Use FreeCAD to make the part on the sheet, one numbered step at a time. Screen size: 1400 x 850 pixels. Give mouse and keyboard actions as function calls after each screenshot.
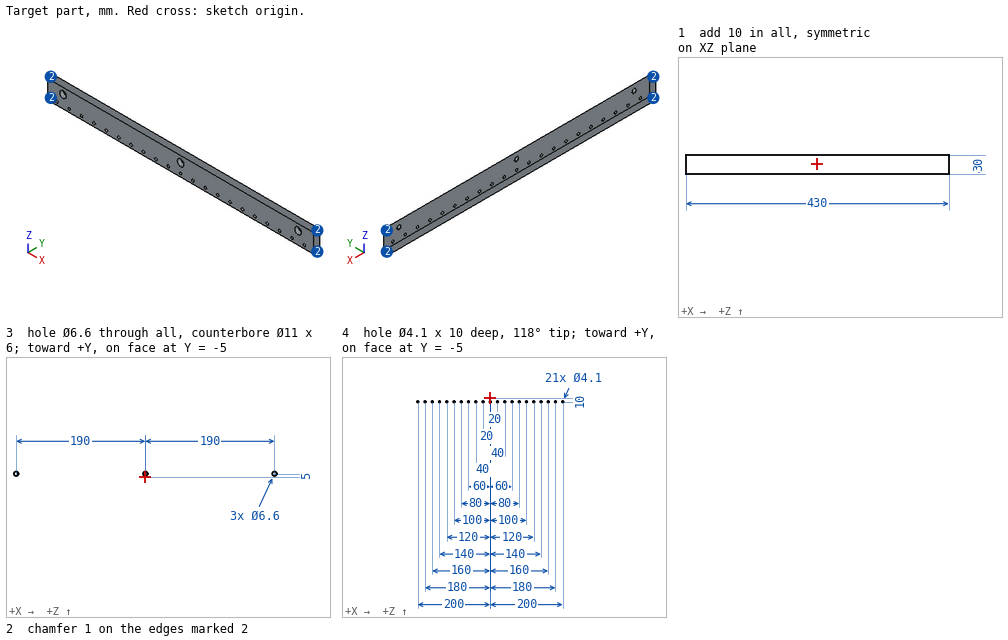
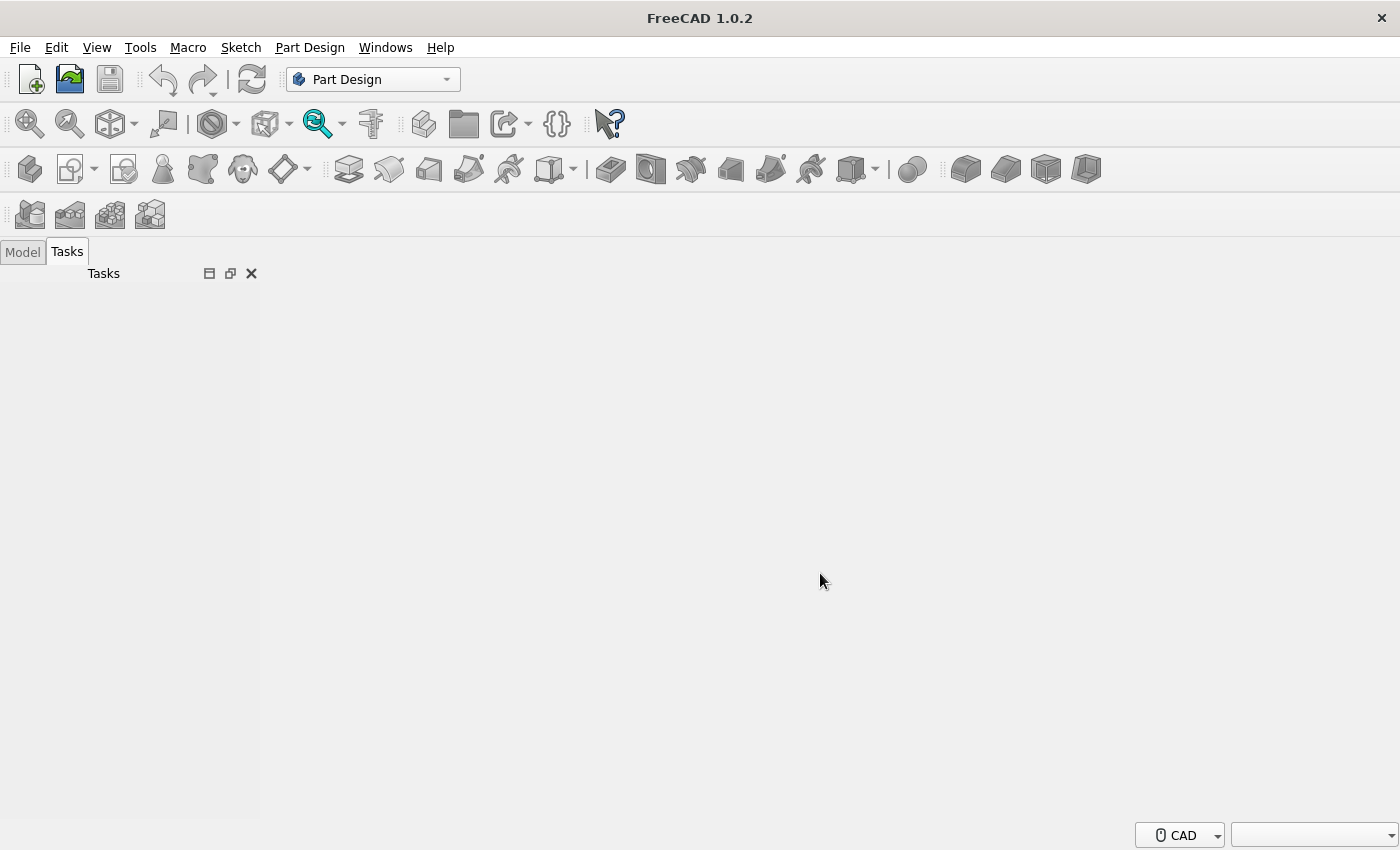
click(30, 80)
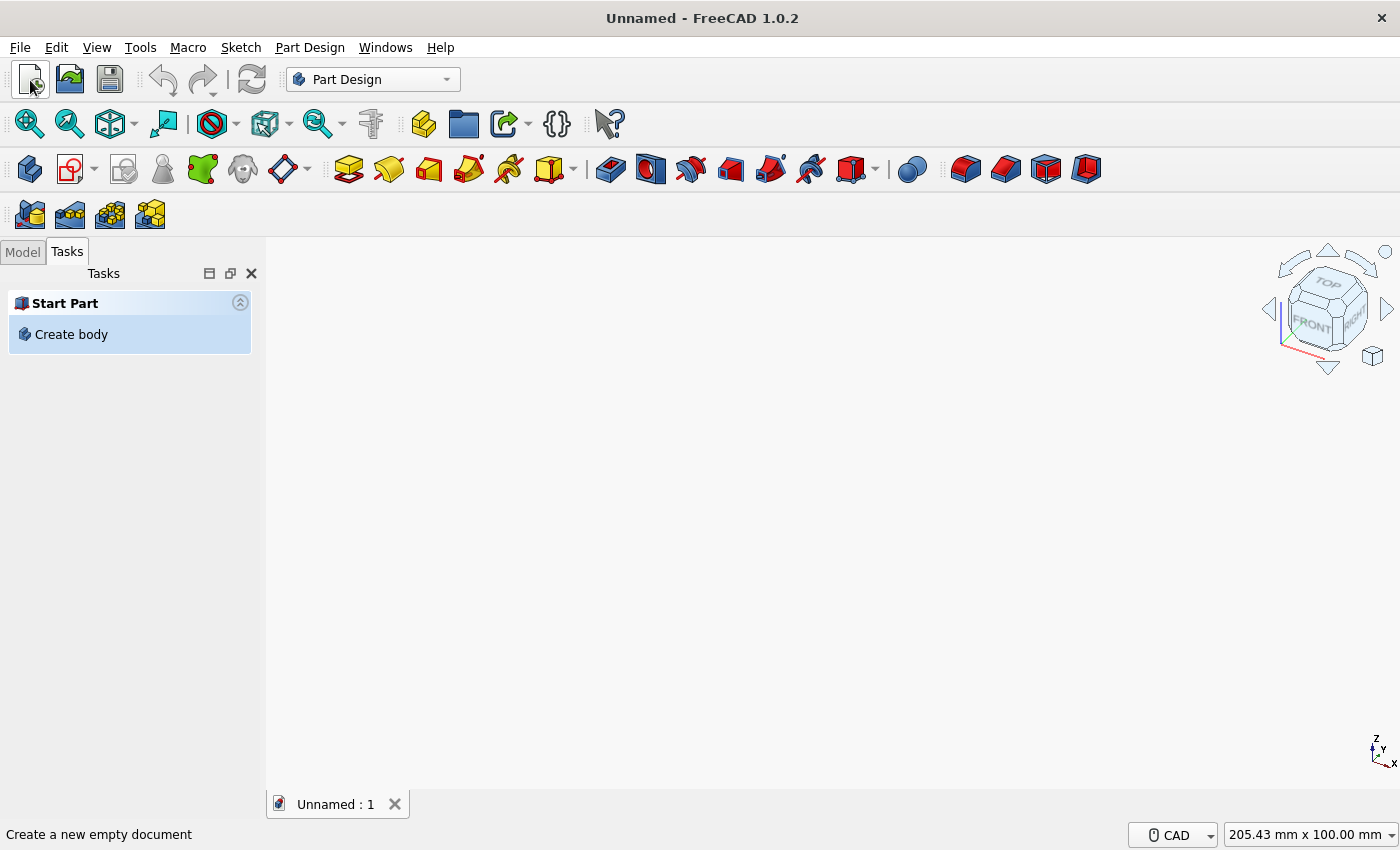
click(70, 170)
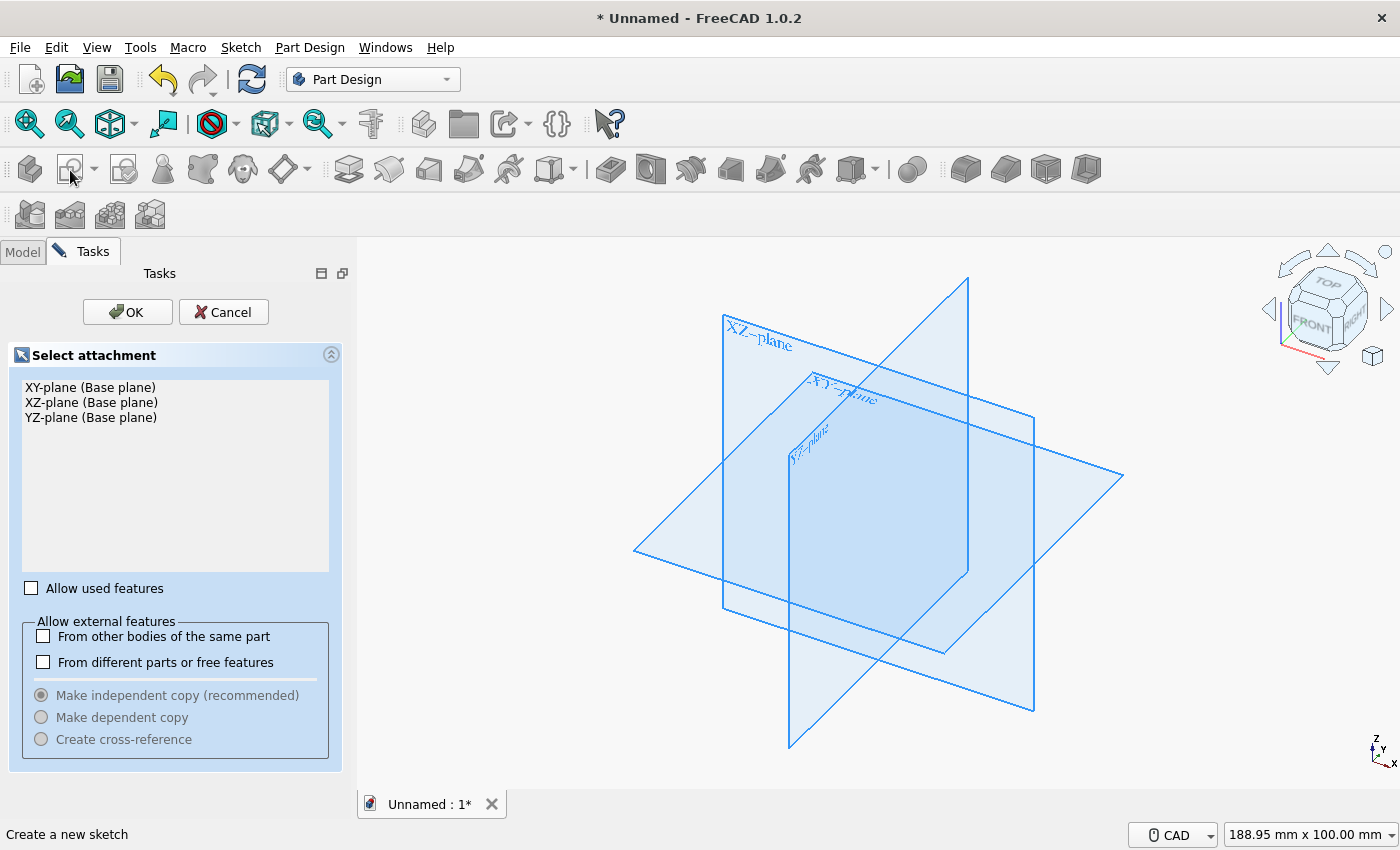
click(82, 402)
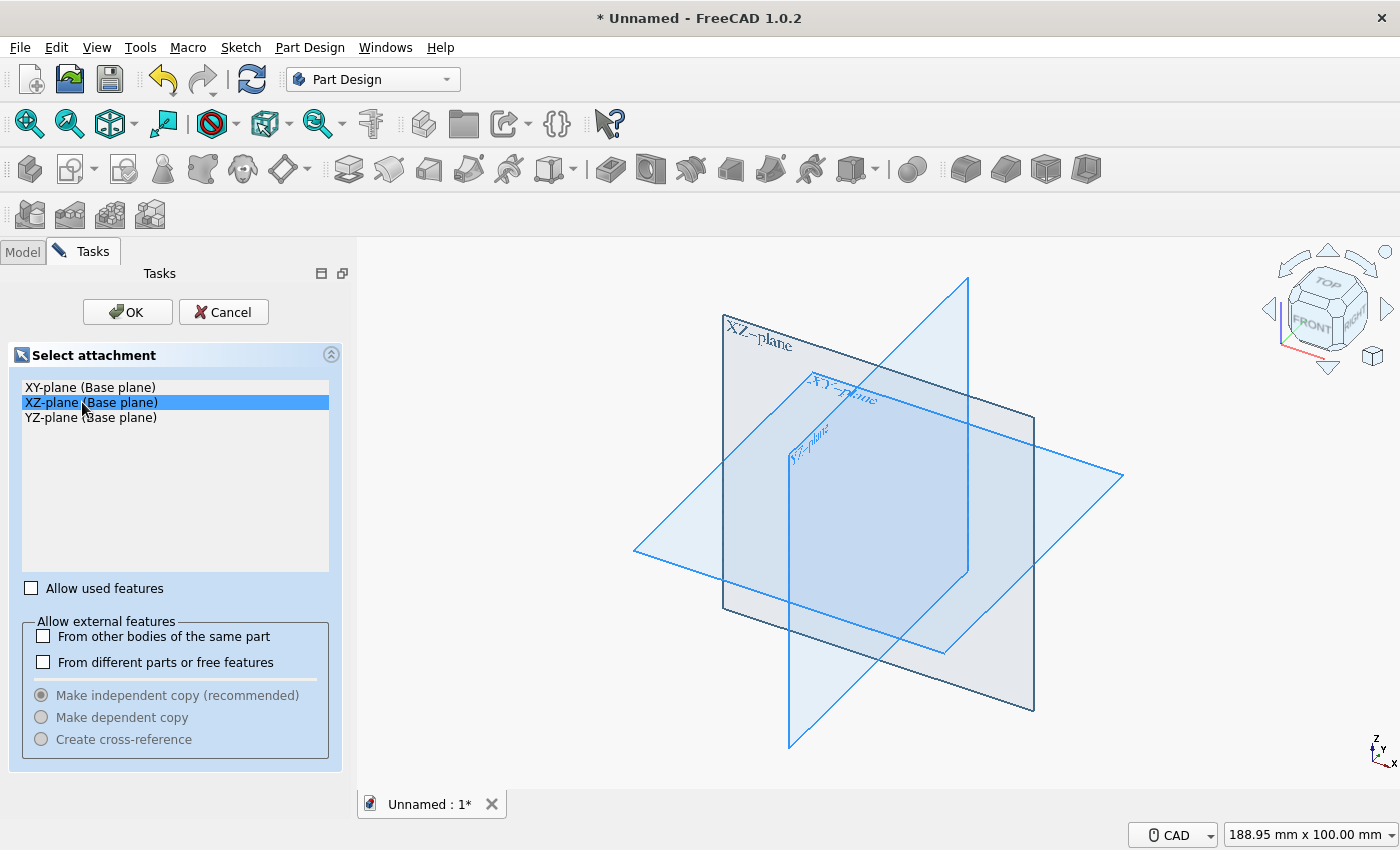
click(128, 312)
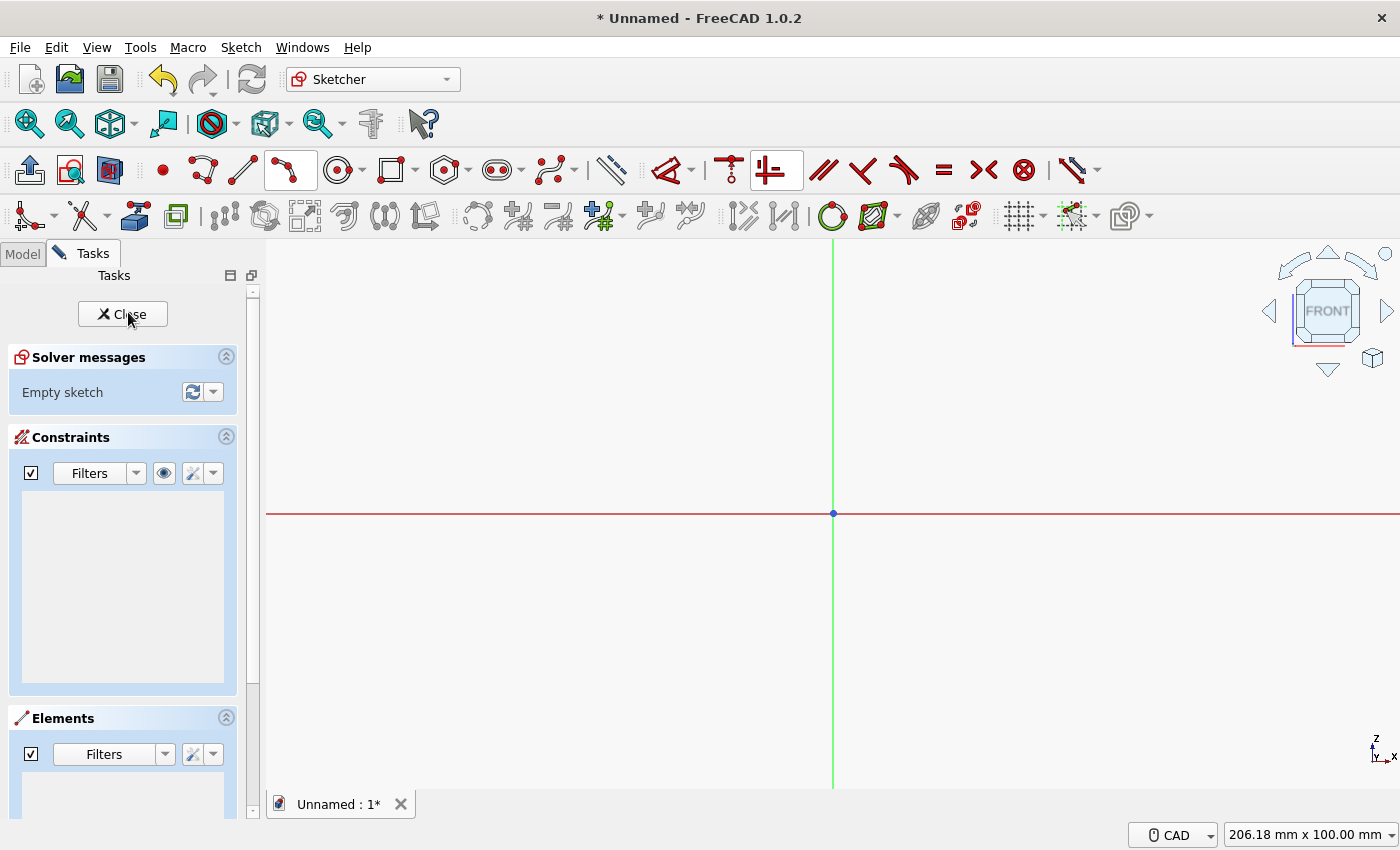
scroll(735, 514, down, 6)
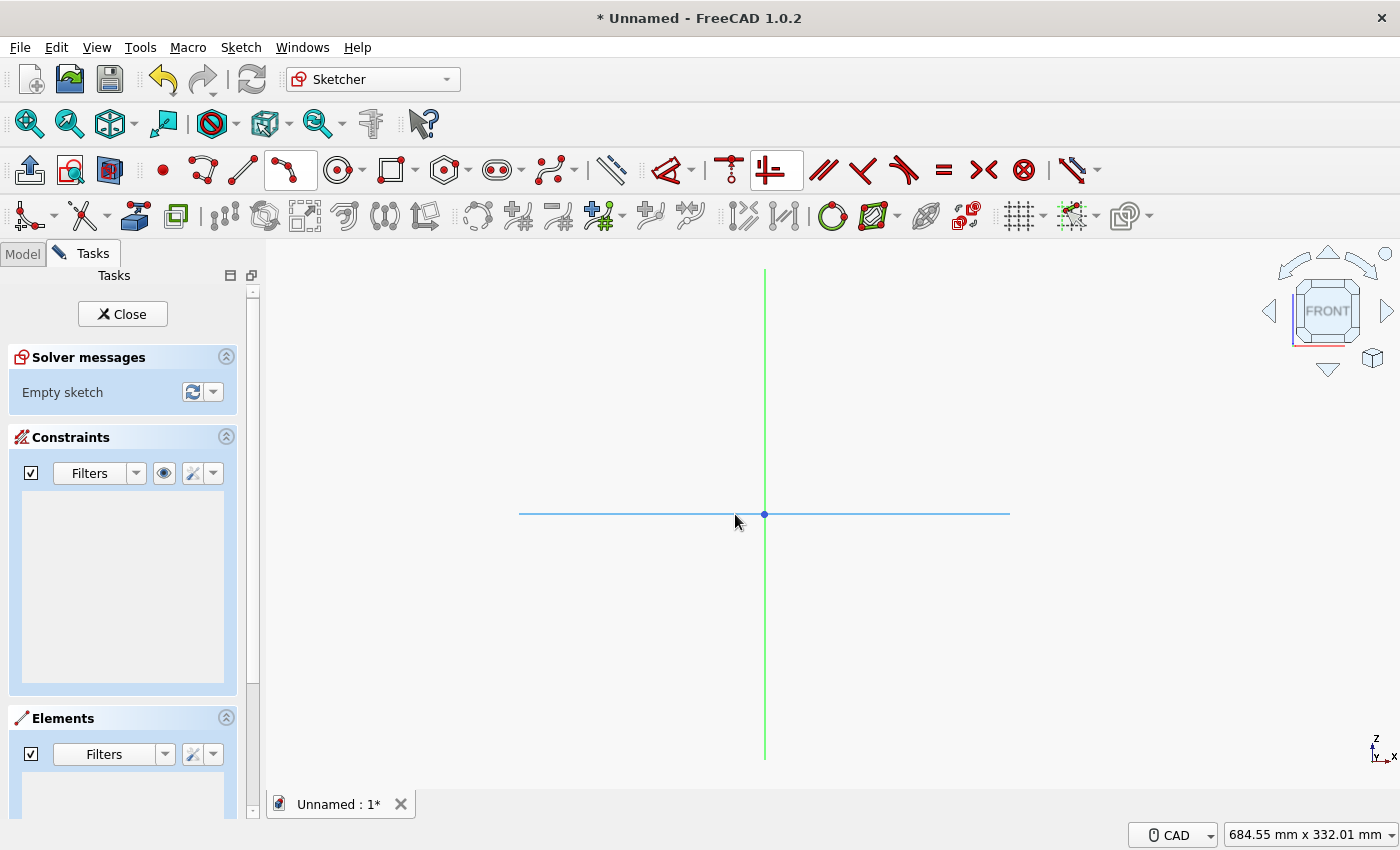
key(g)
key(v)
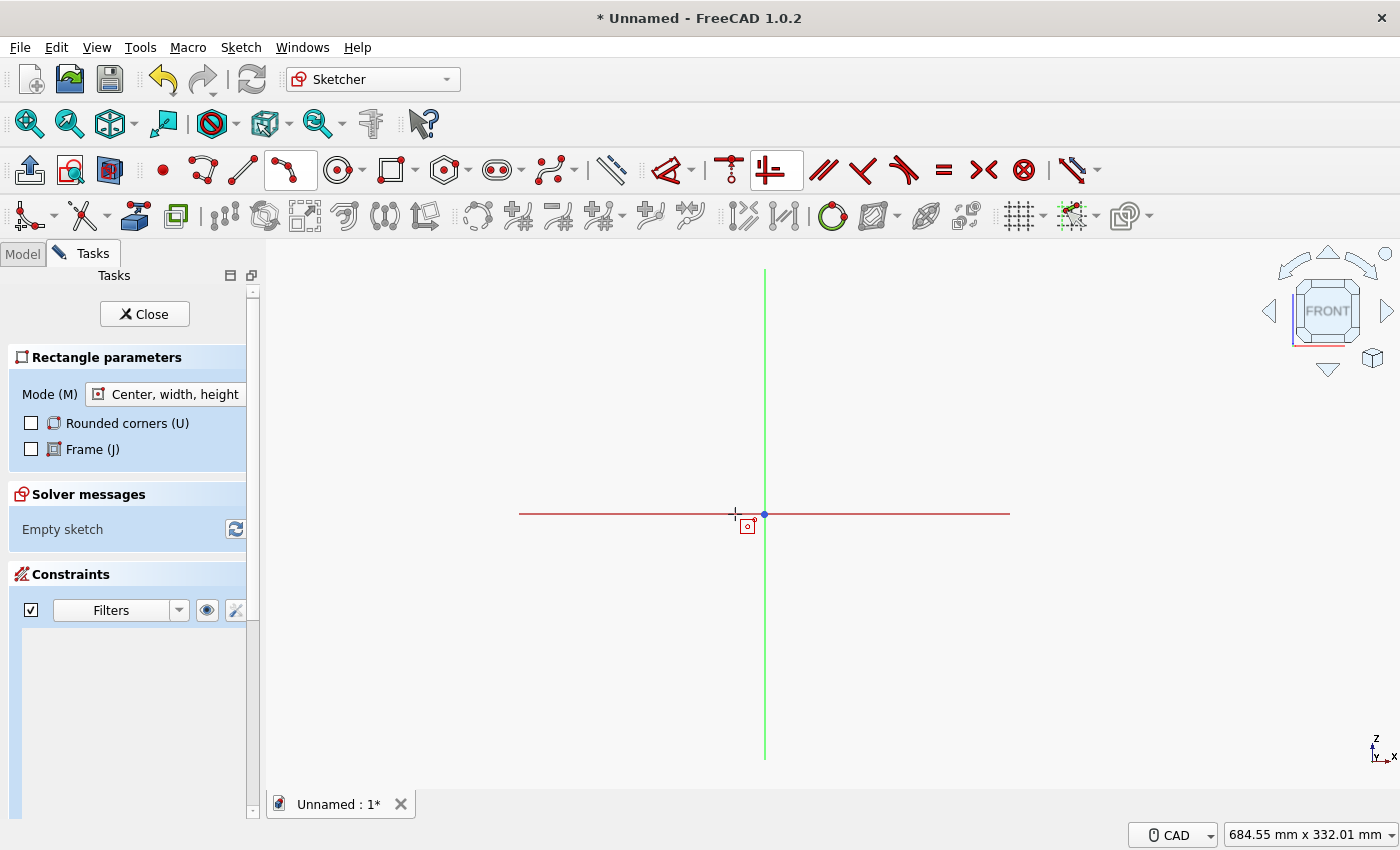
click(765, 514)
click(1121, 490)
key(Escape)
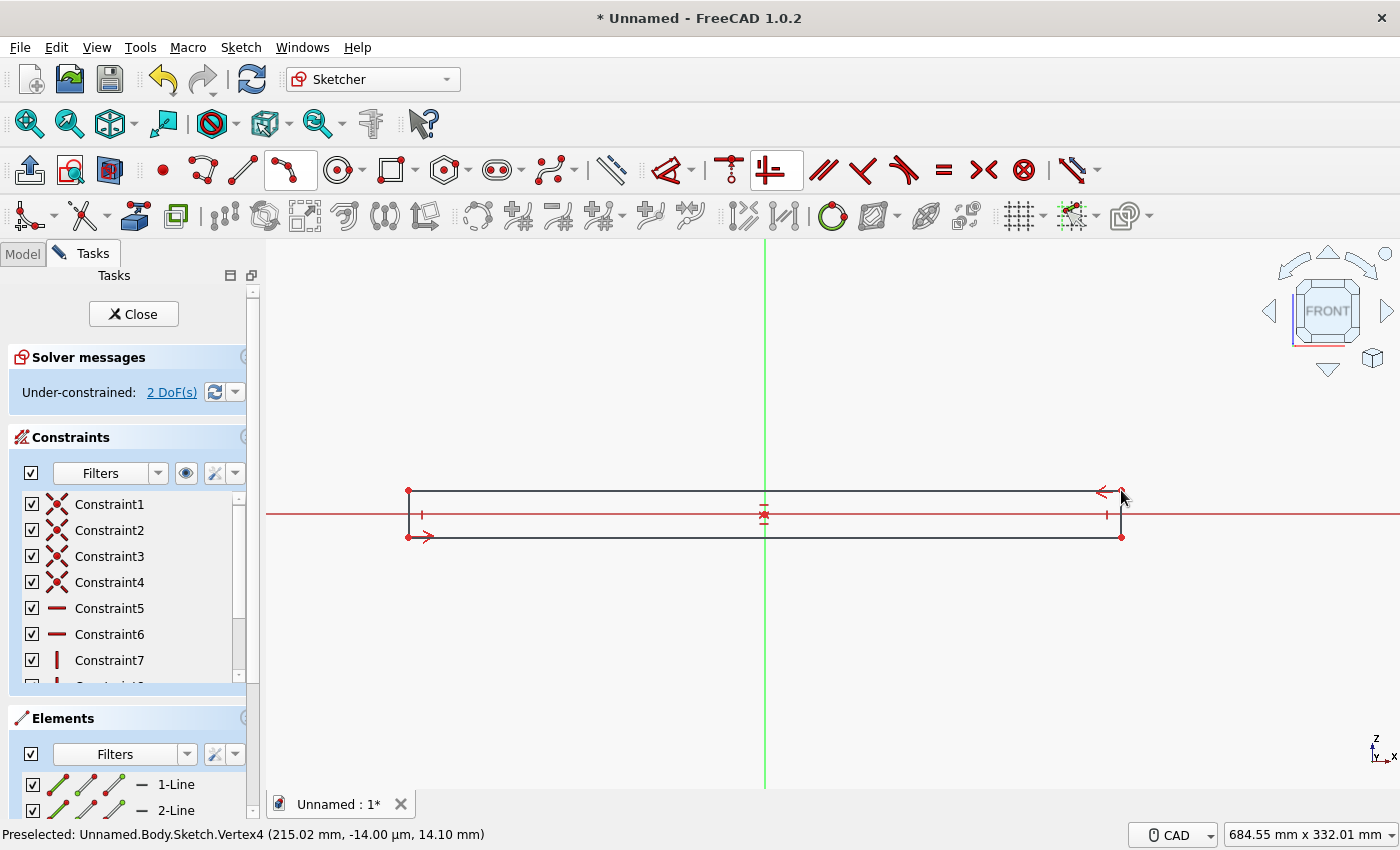
scroll(1121, 524, up, 2)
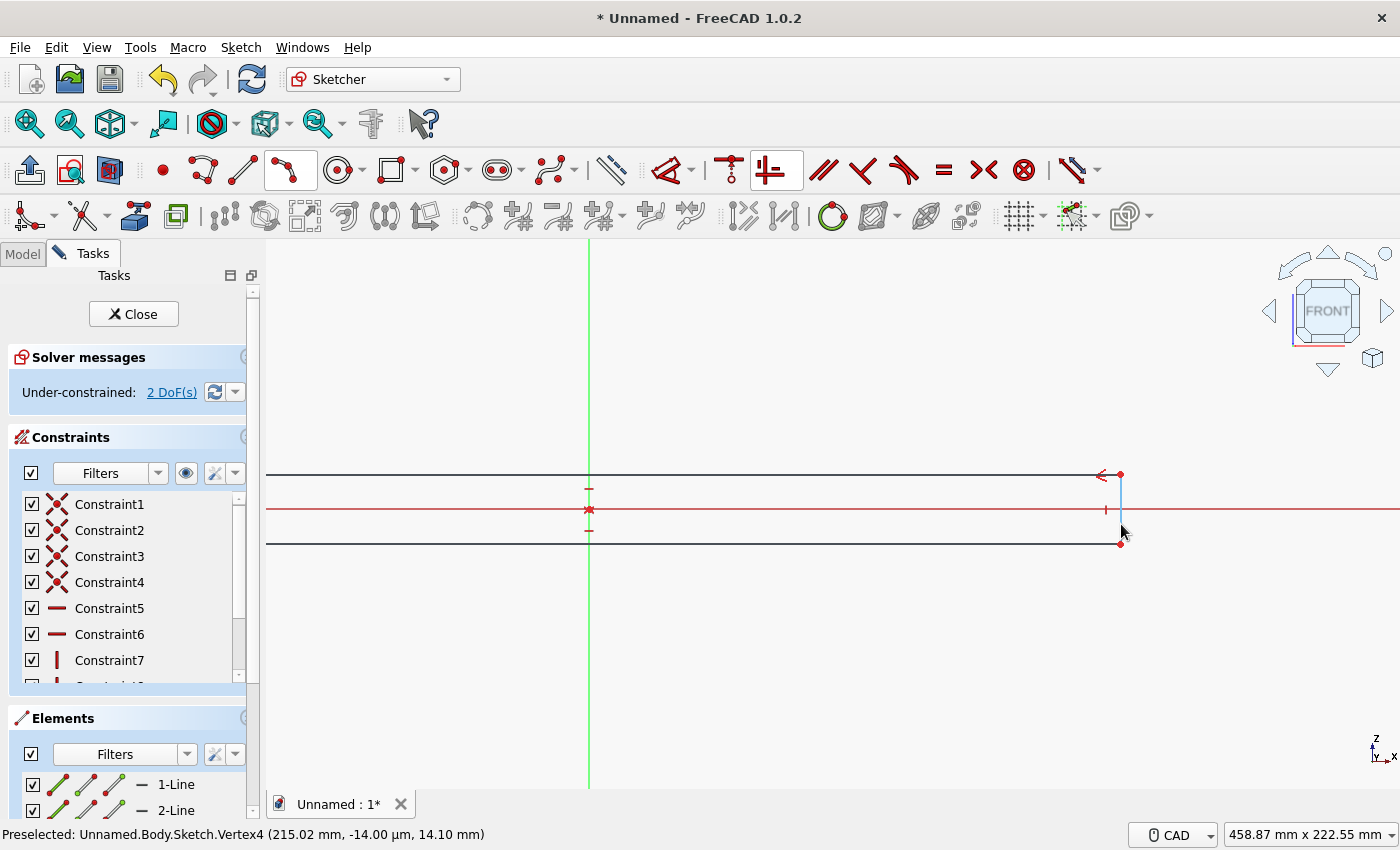
click(1121, 523)